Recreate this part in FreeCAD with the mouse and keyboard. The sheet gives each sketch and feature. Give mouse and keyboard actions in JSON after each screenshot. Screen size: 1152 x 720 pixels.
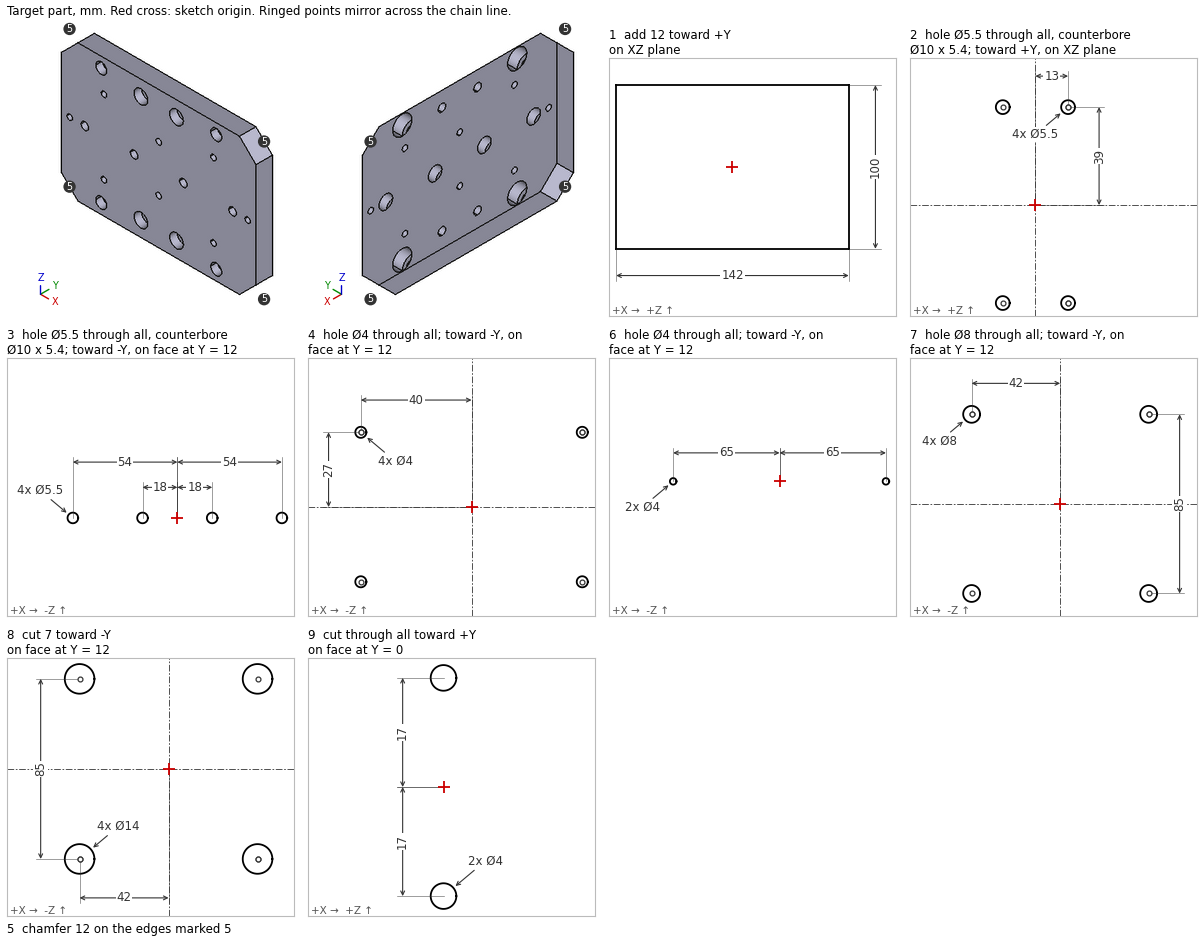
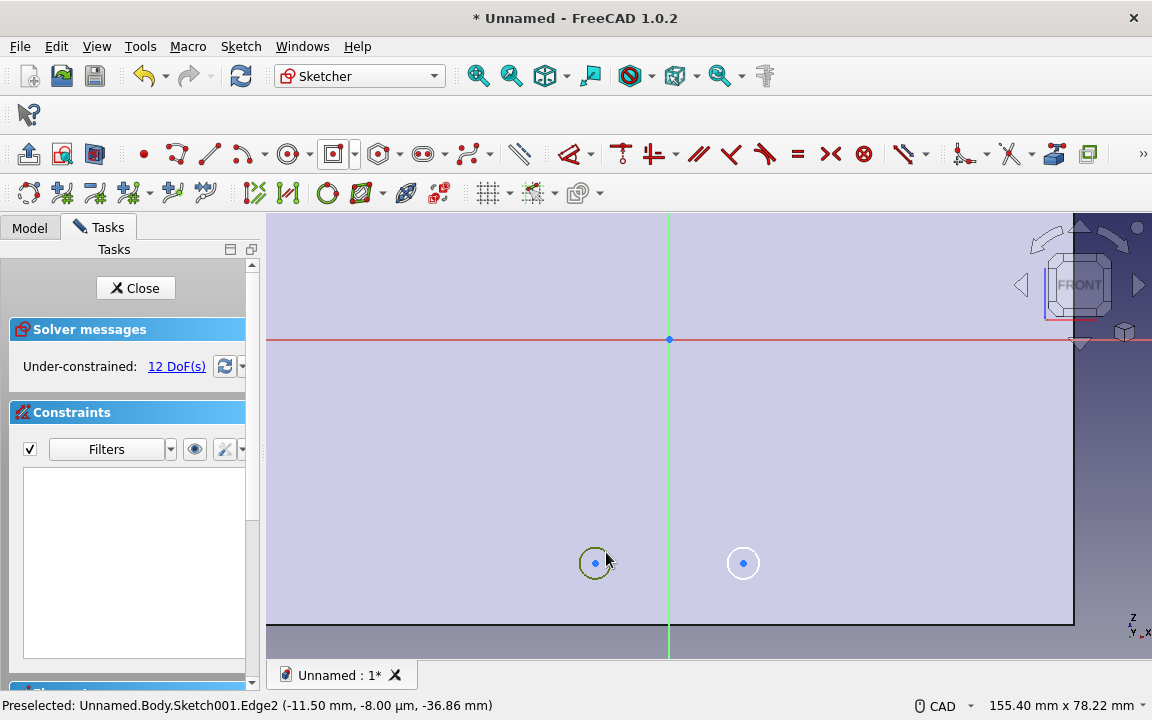
{"action": "left_click", "coordinate": [754, 552]}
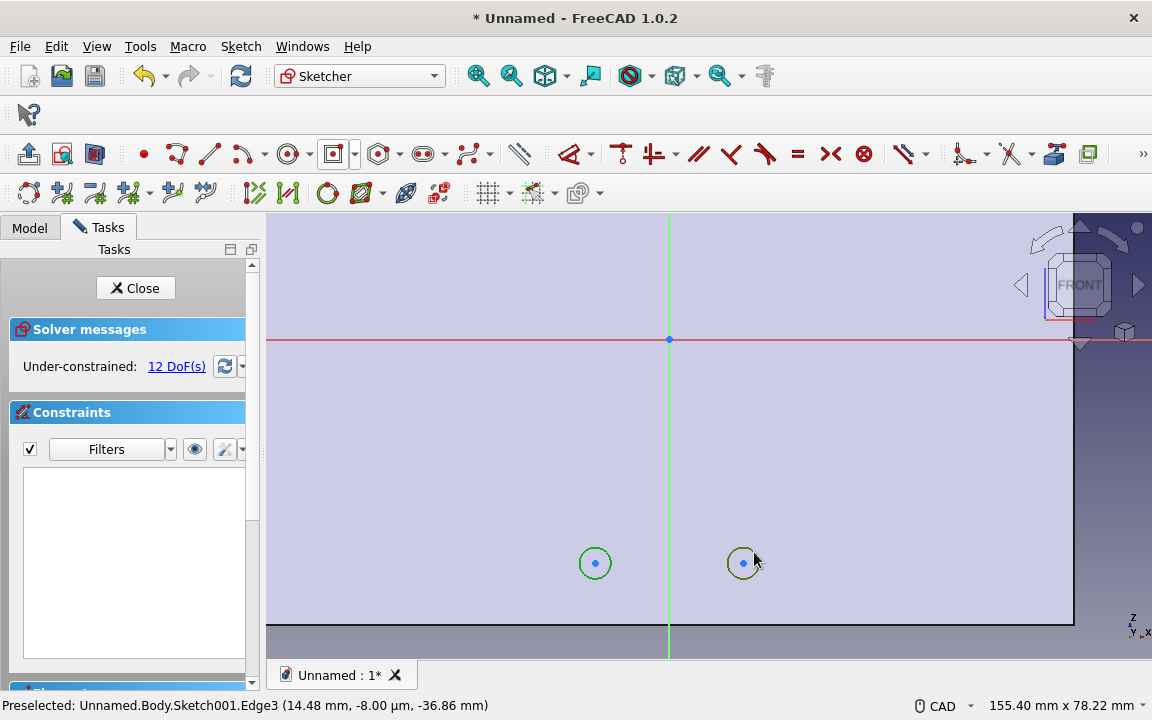
{"action": "scroll", "coordinate": [606, 553], "scroll_direction": "down", "scroll_amount": 3}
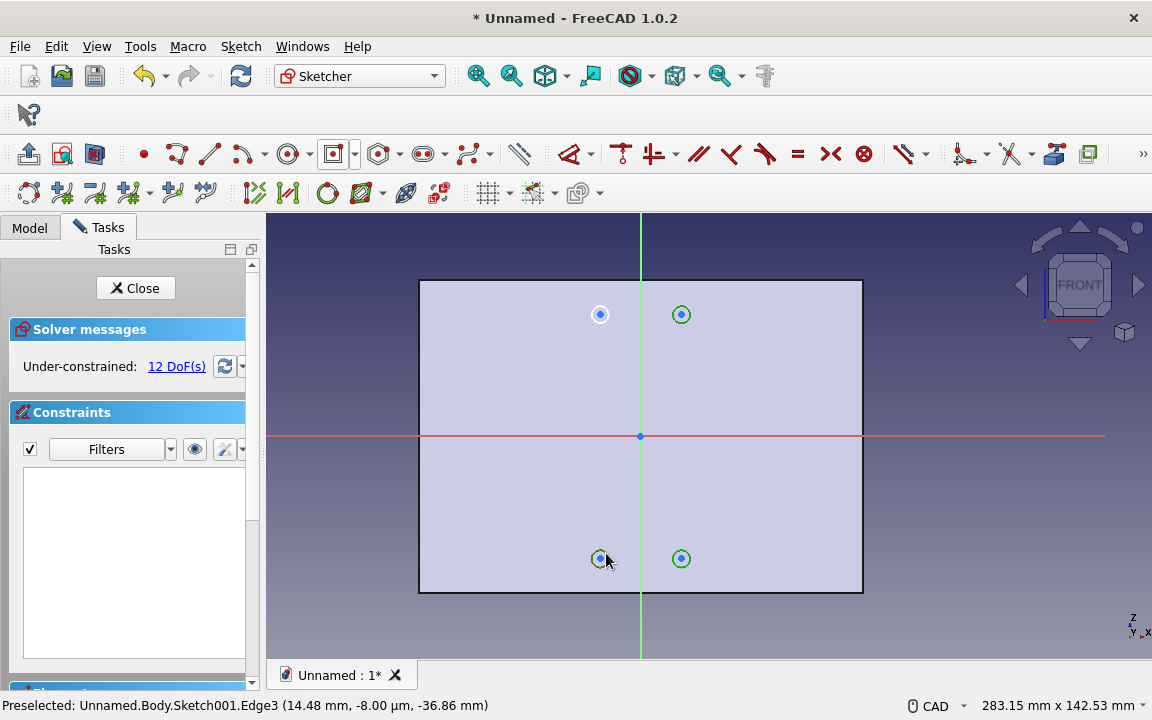
{"action": "scroll", "coordinate": [606, 309], "scroll_direction": "up", "scroll_amount": 3}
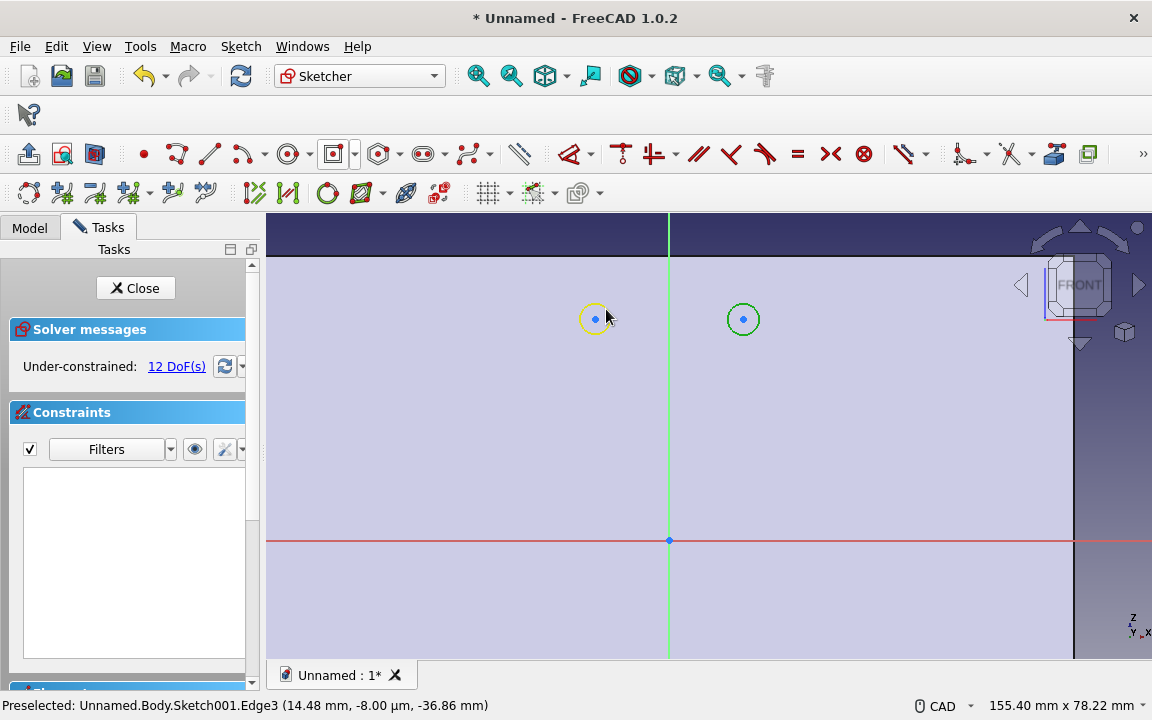
{"action": "left_click", "coordinate": [606, 308]}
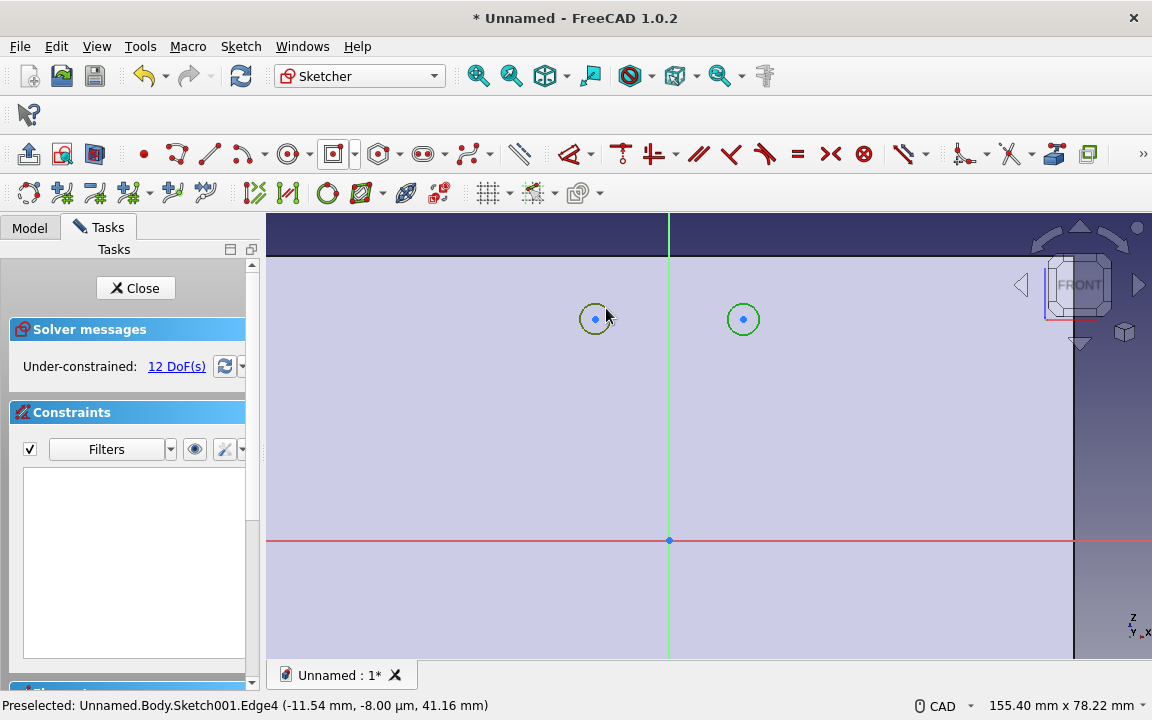
{"action": "left_click", "coordinate": [798, 154]}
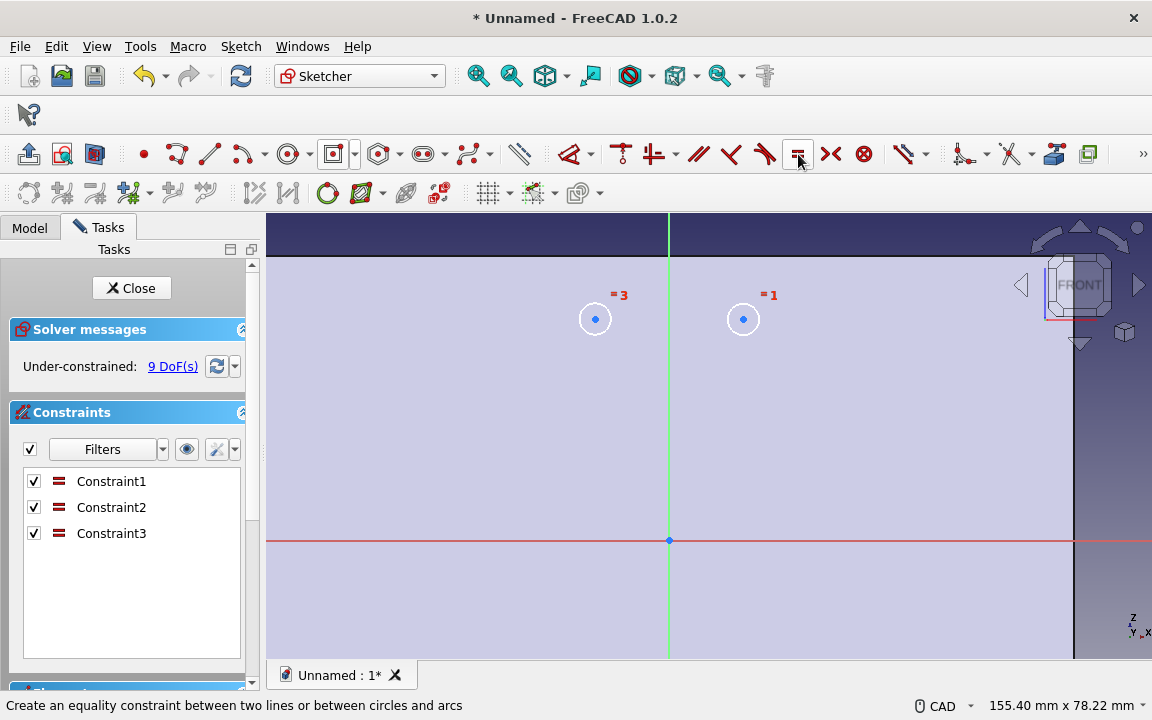
{"action": "left_click", "coordinate": [743, 319]}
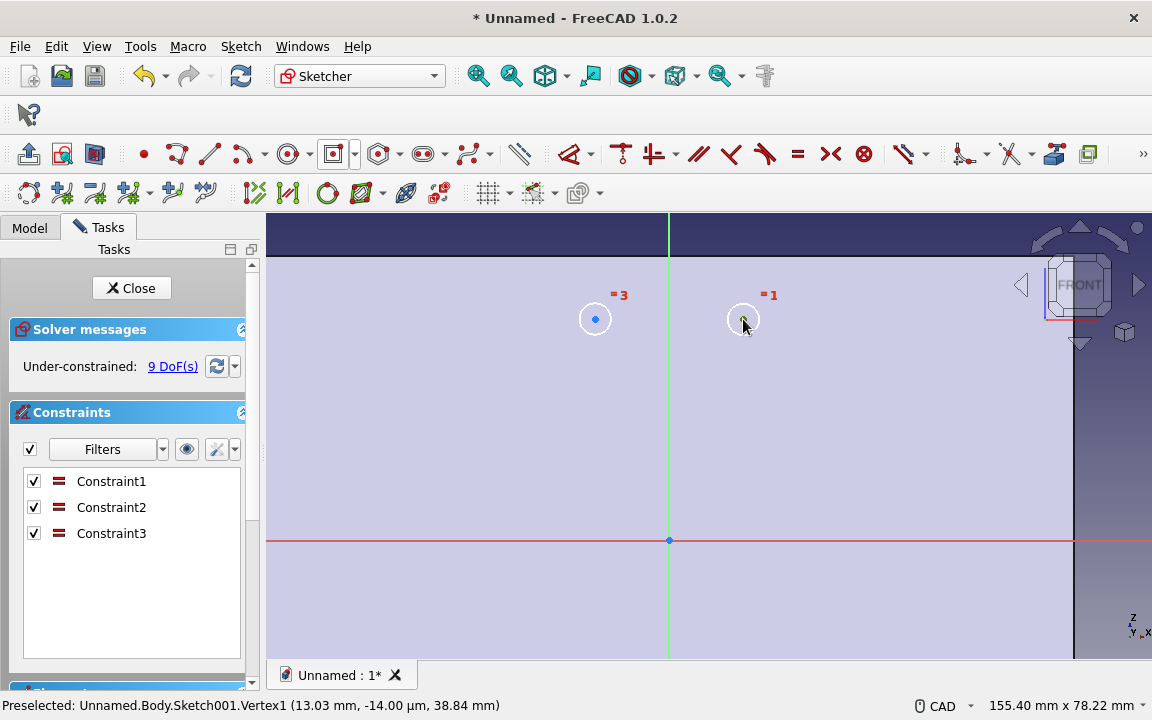
{"action": "scroll", "coordinate": [606, 308], "scroll_direction": "down", "scroll_amount": 3}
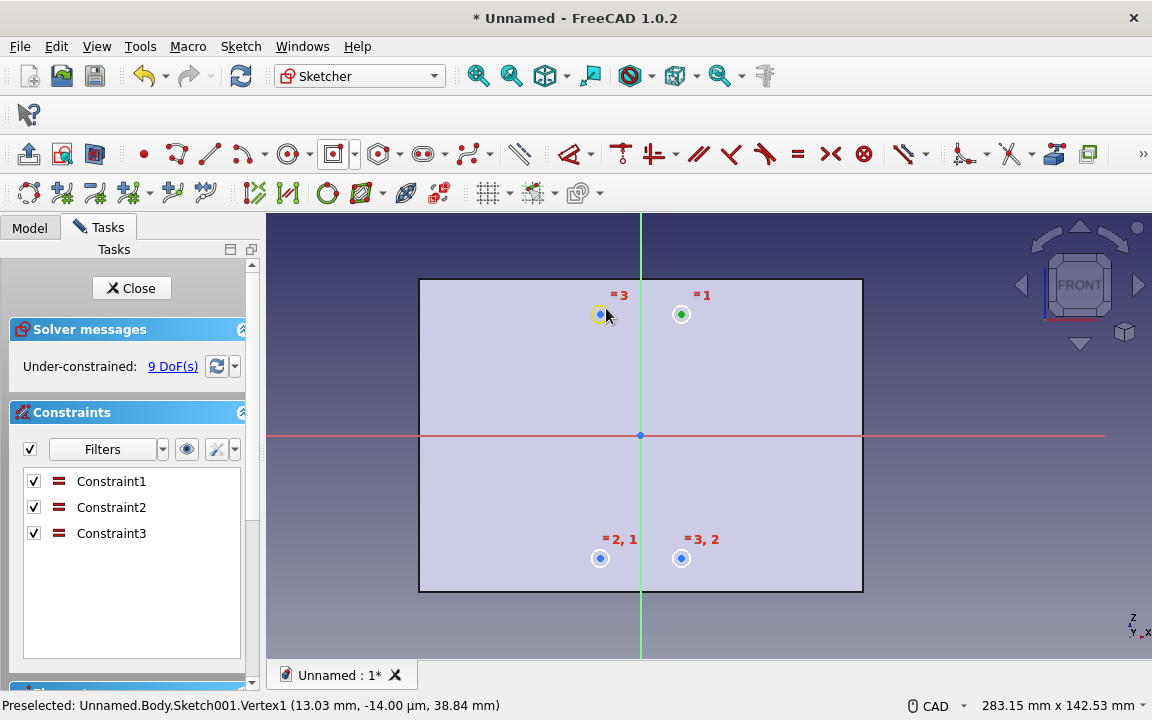
{"action": "left_click", "coordinate": [682, 558]}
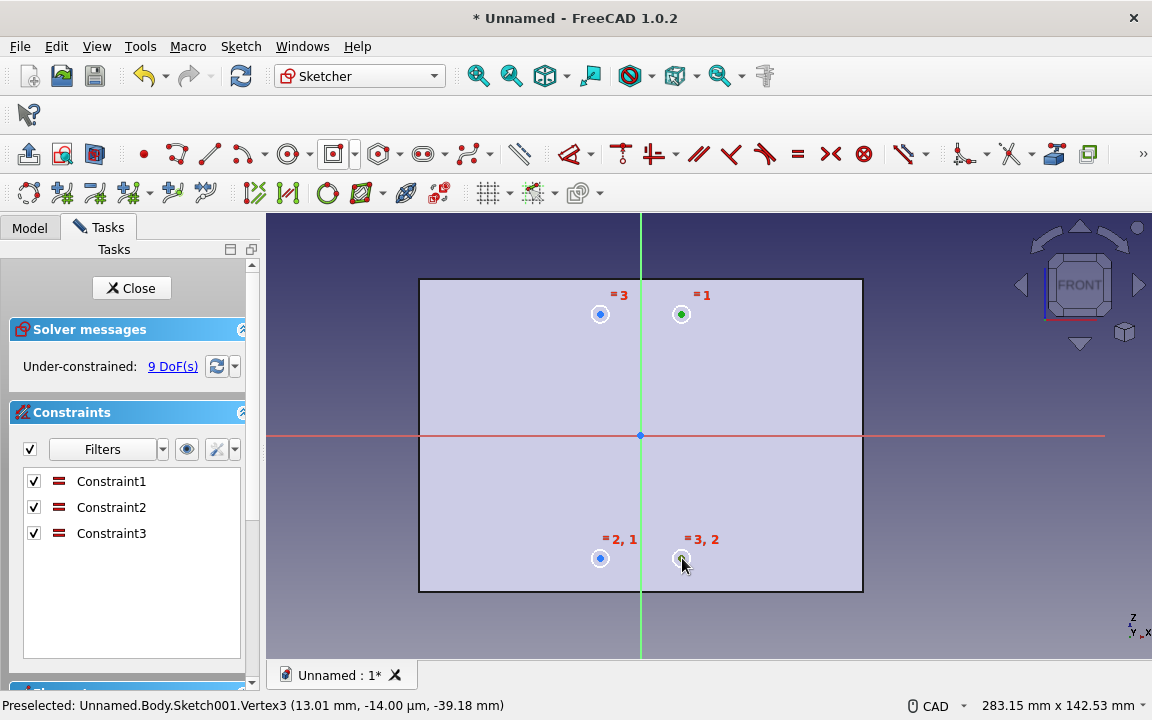
{"action": "left_click", "coordinate": [344, 436]}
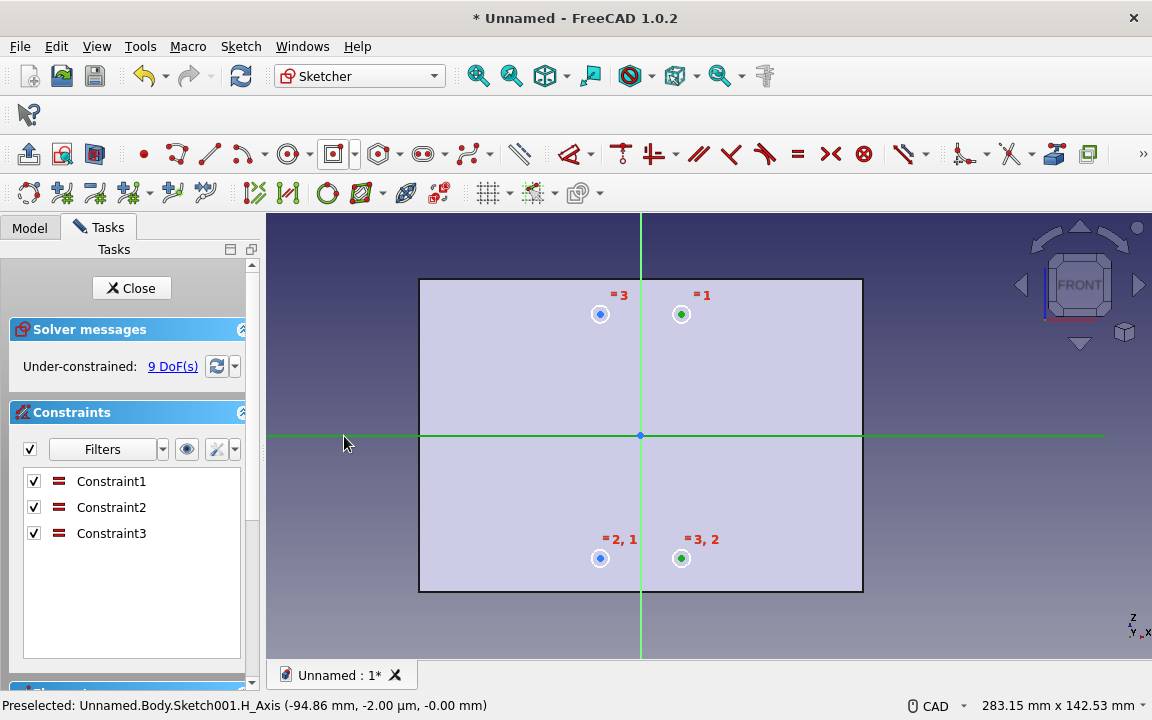
{"action": "left_click", "coordinate": [831, 154]}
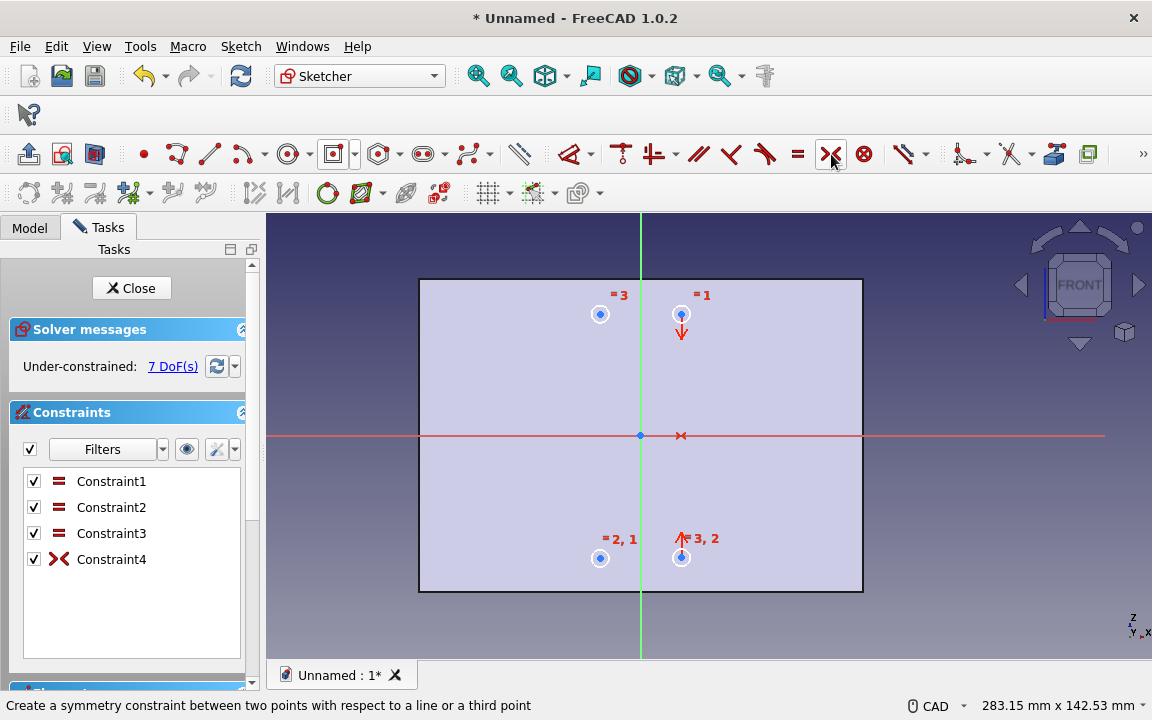
{"action": "left_click", "coordinate": [600, 558]}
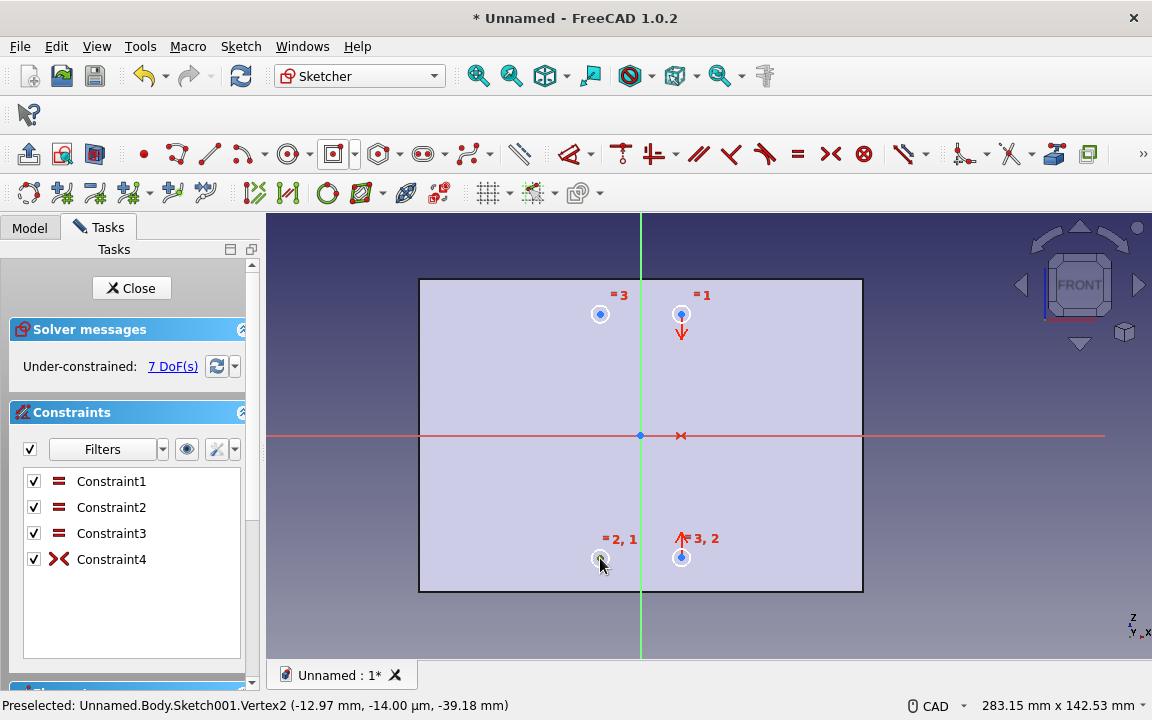
{"action": "left_click", "coordinate": [682, 558]}